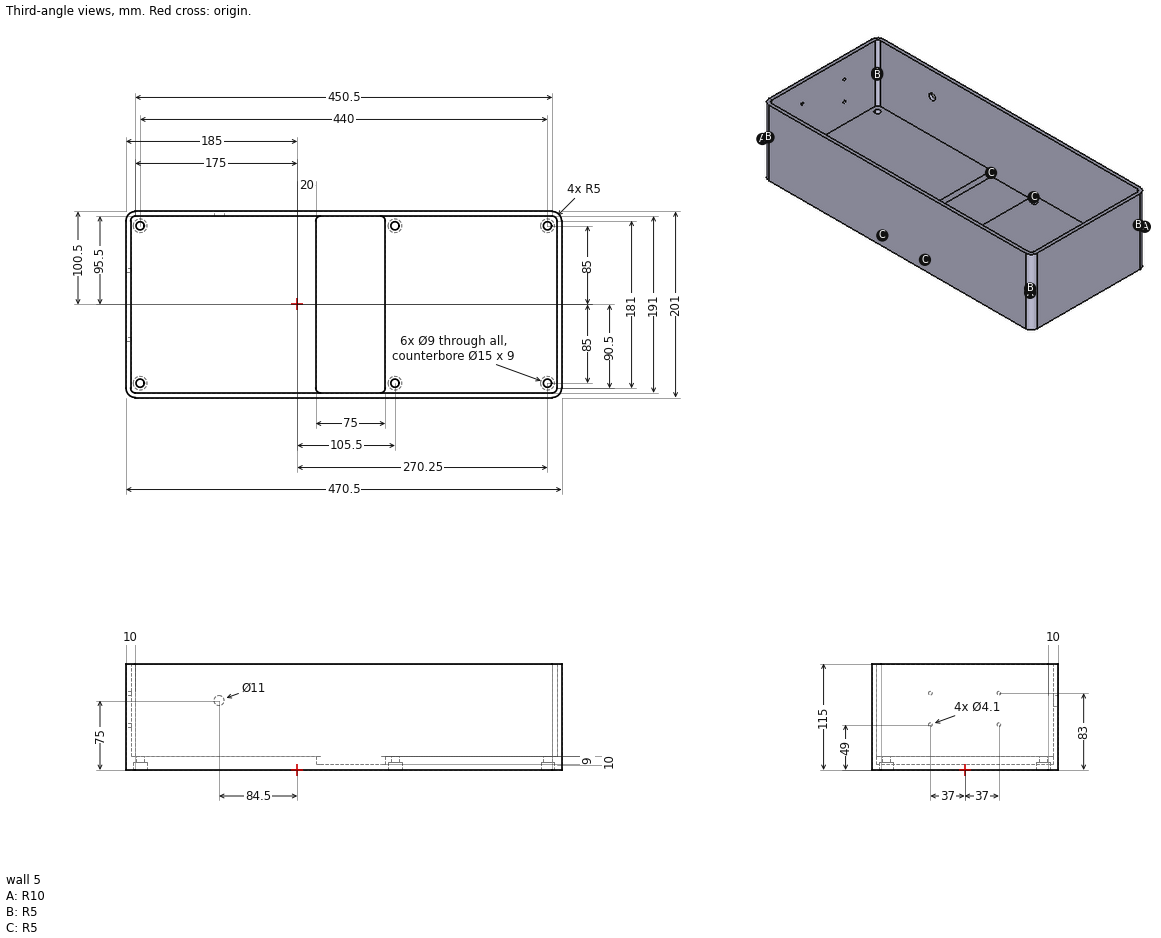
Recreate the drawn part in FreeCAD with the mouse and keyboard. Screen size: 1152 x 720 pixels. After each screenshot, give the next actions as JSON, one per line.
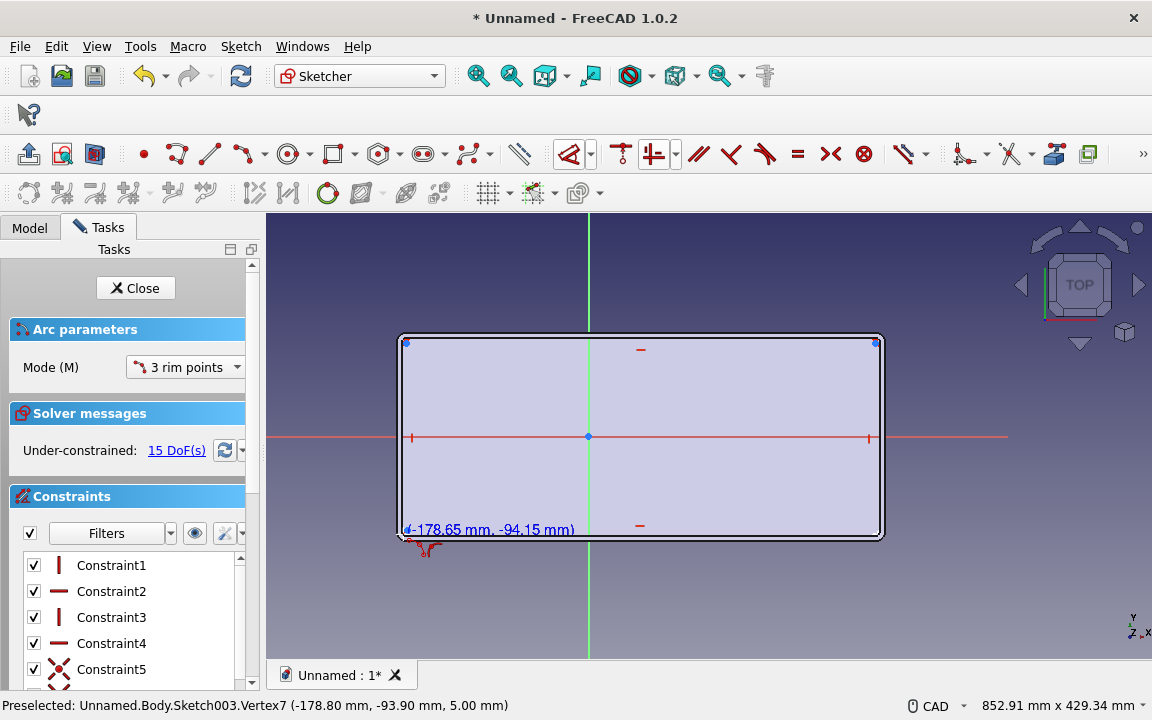
{"action": "scroll", "coordinate": [875, 536], "scroll_direction": "up", "scroll_amount": 4}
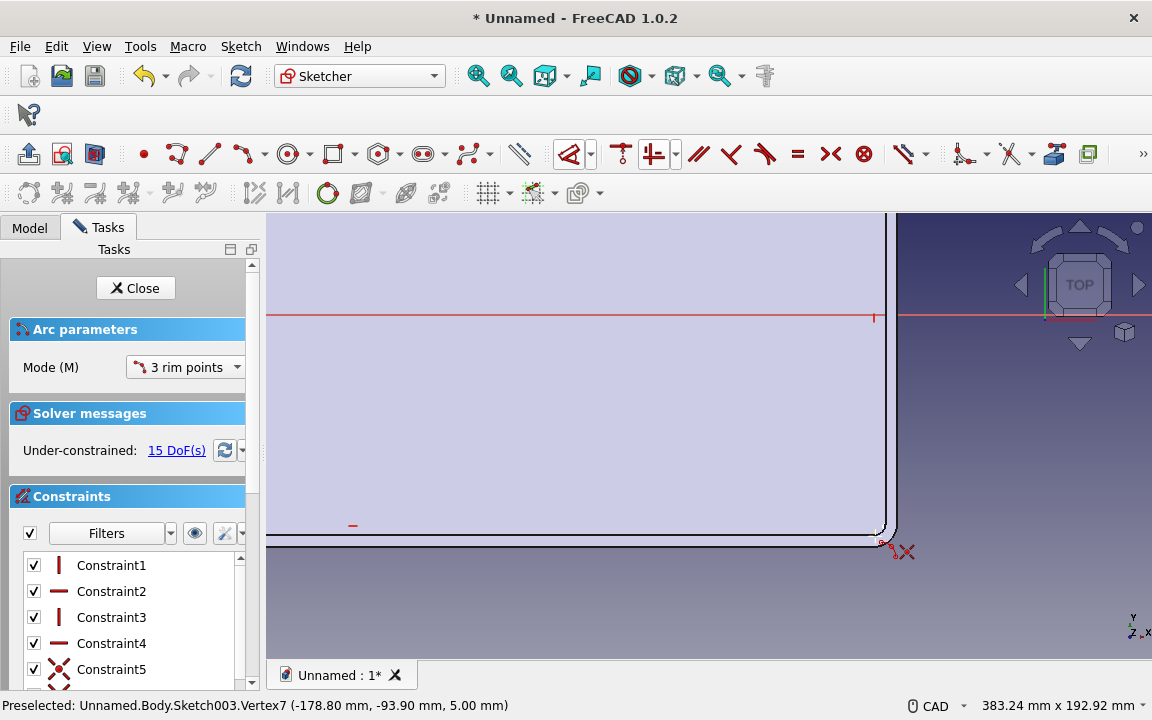
{"action": "left_click", "coordinate": [874, 536]}
{"action": "left_click", "coordinate": [886, 527]}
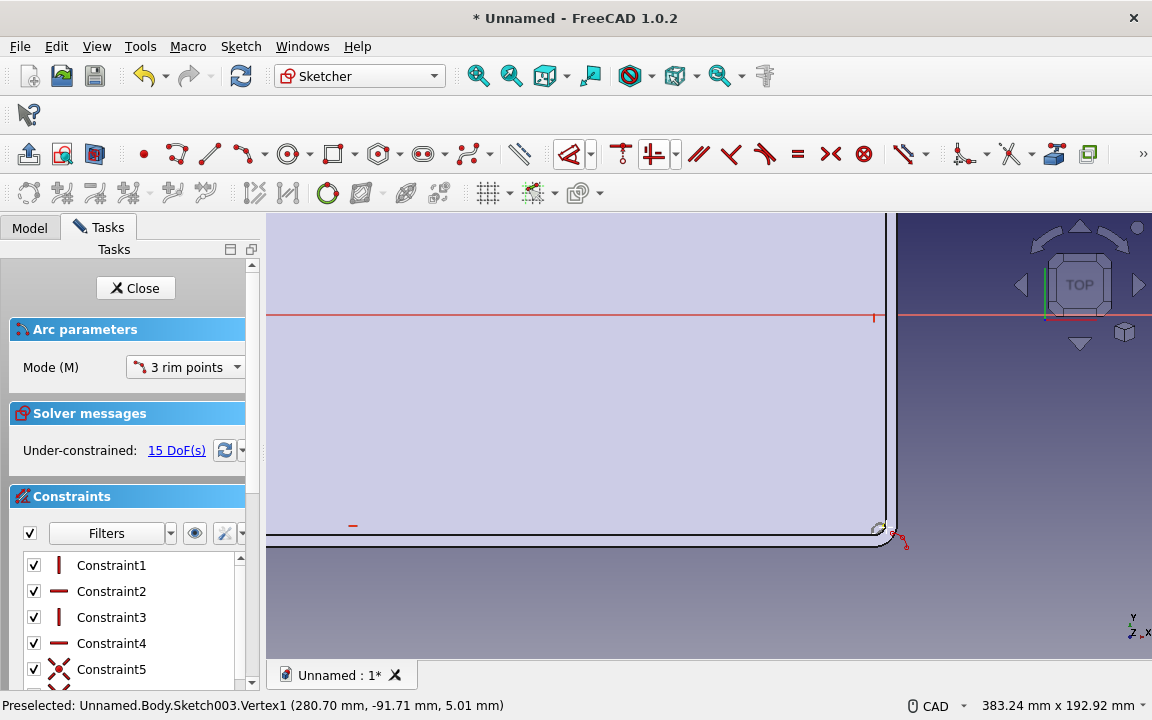
{"action": "scroll", "coordinate": [882, 532], "scroll_direction": "up", "scroll_amount": 8}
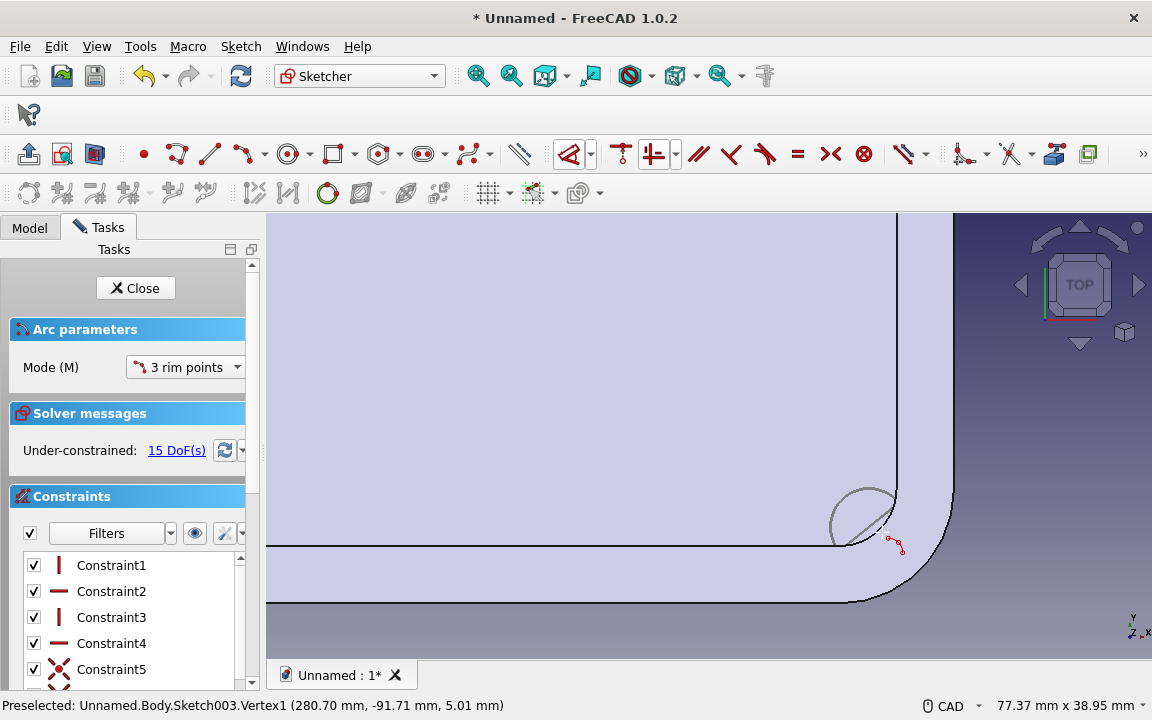
{"action": "left_click", "coordinate": [880, 529]}
{"action": "key", "text": "Escape"}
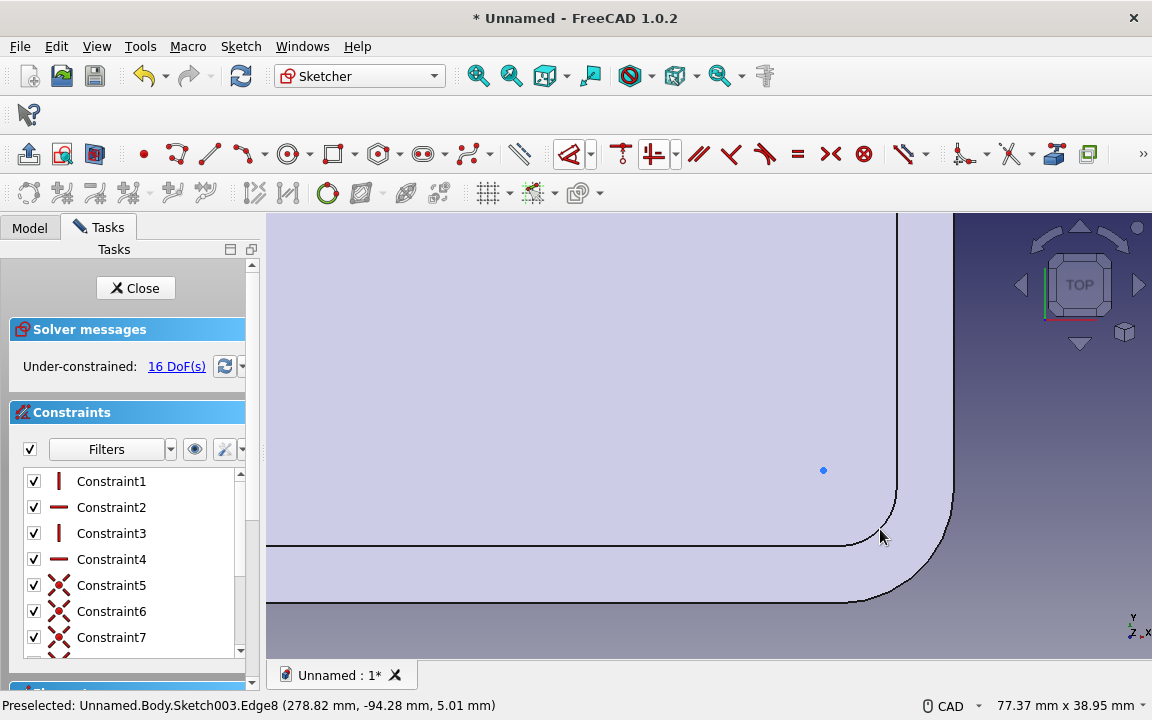
{"action": "scroll", "coordinate": [878, 534], "scroll_direction": "down", "scroll_amount": 12}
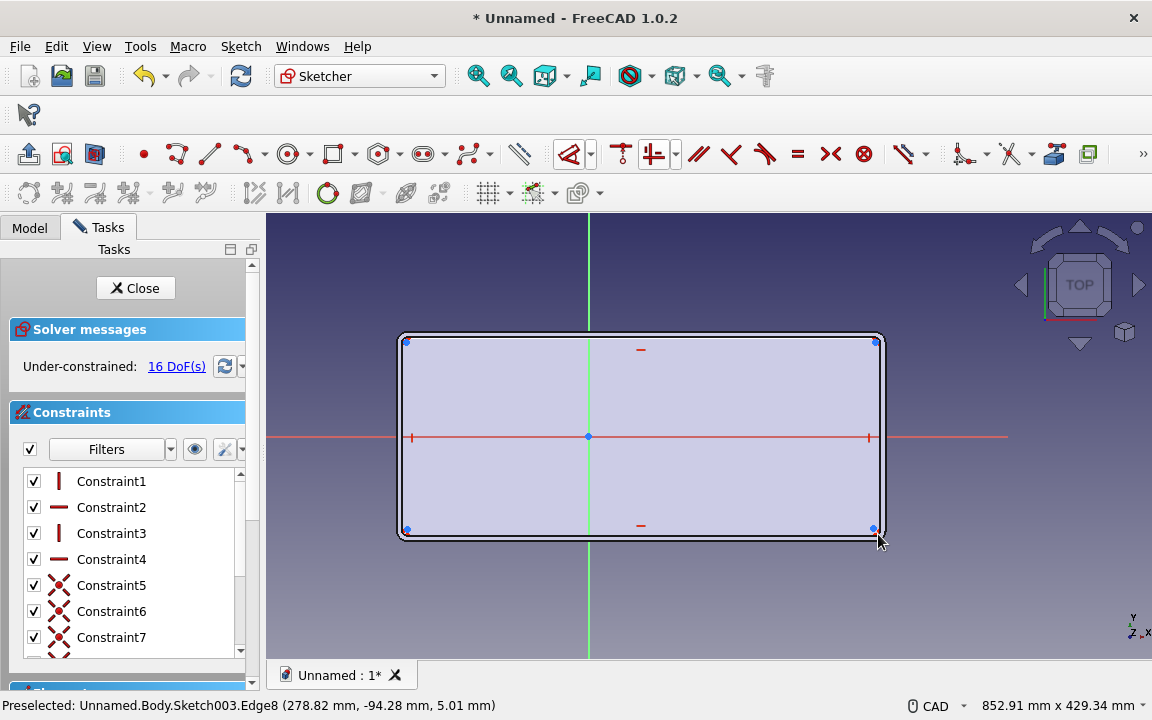
{"action": "left_click", "coordinate": [881, 475]}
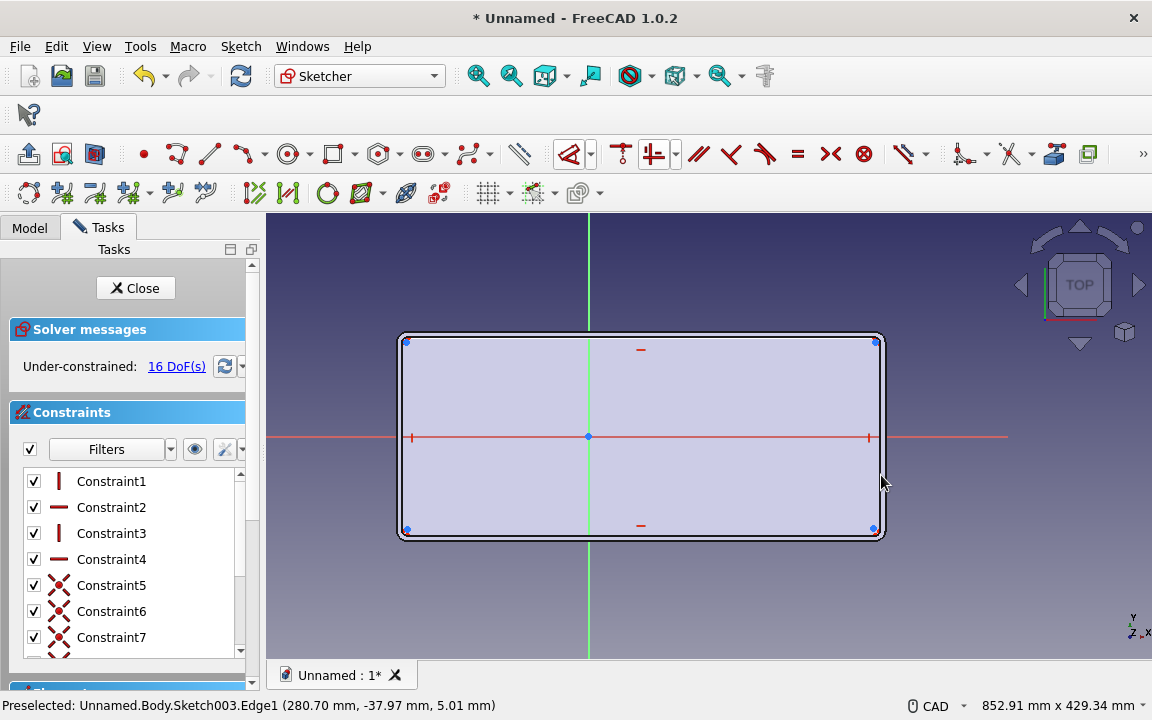
{"action": "scroll", "coordinate": [879, 339], "scroll_direction": "up", "scroll_amount": 6}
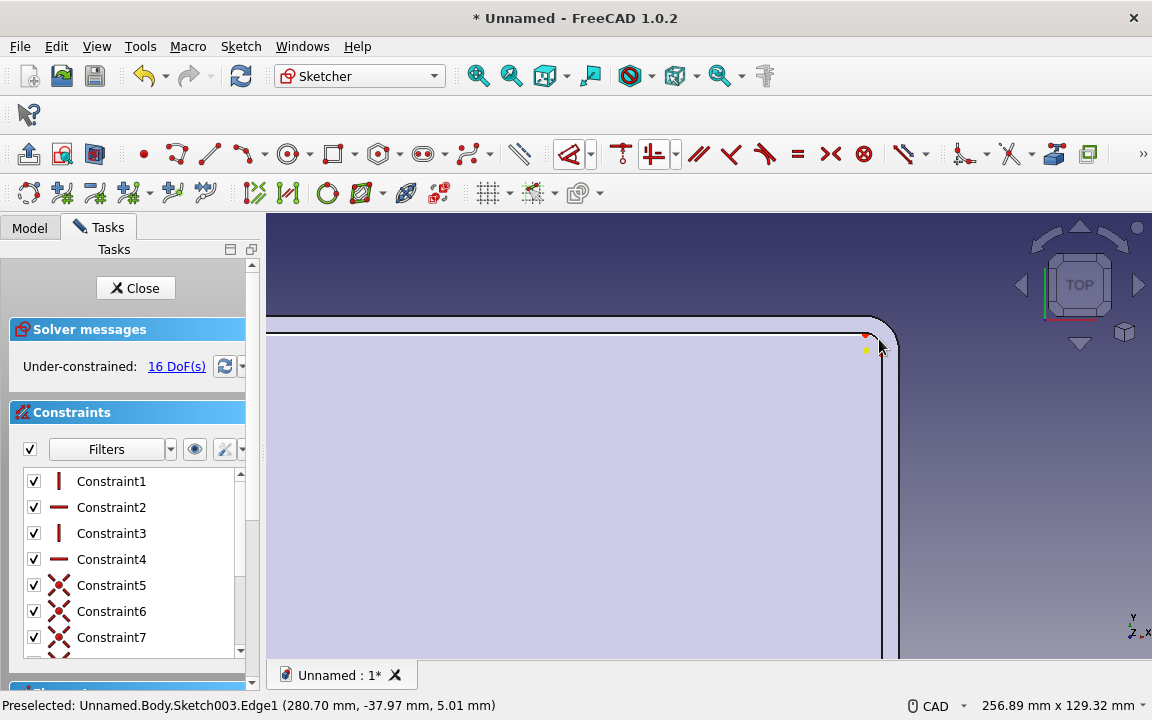
{"action": "left_click", "coordinate": [879, 340]}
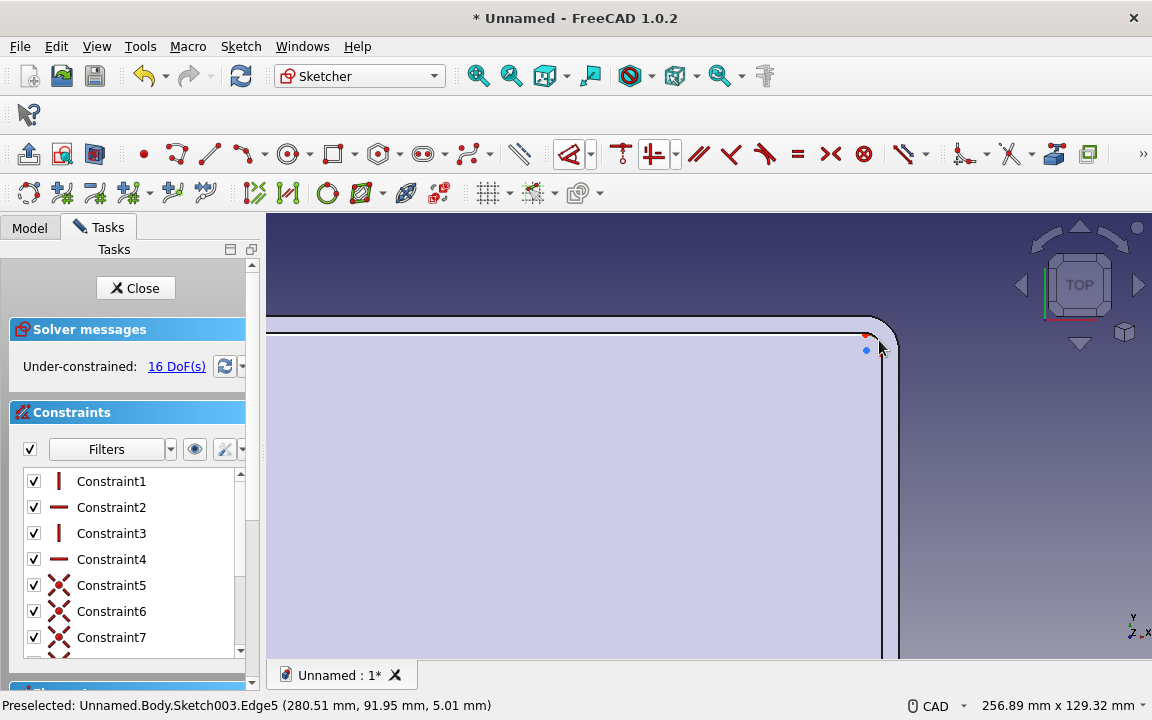
{"action": "key", "text": "t"}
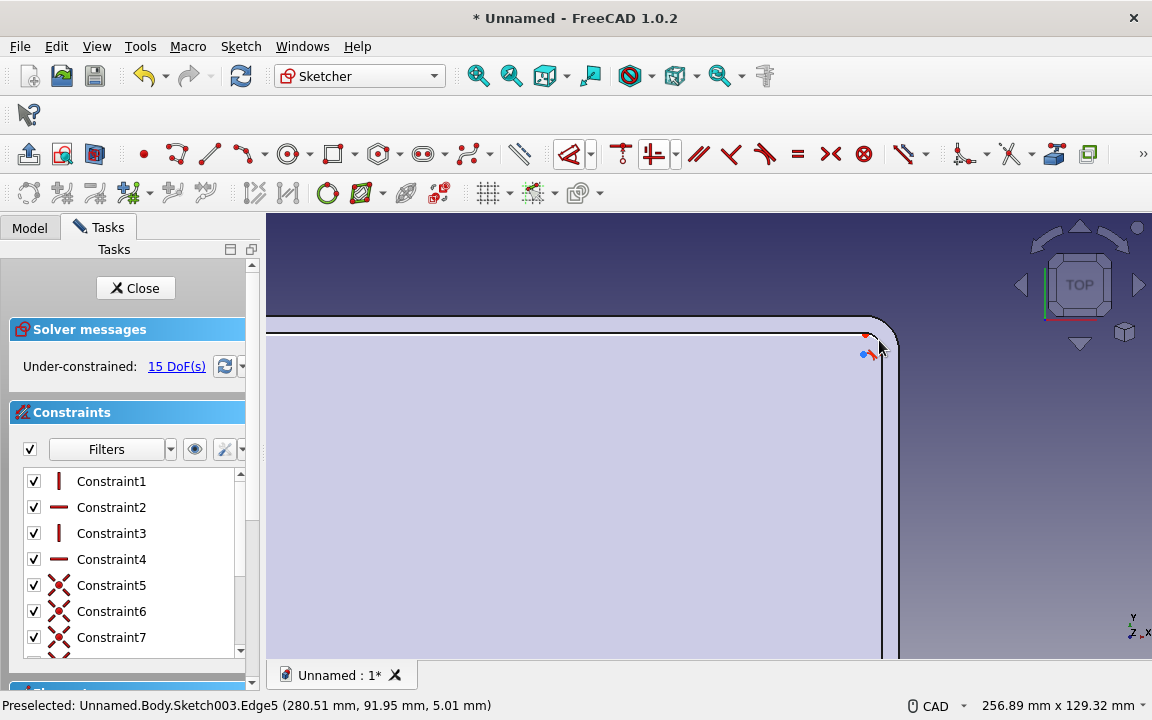
{"action": "scroll", "coordinate": [879, 338], "scroll_direction": "down", "scroll_amount": 6}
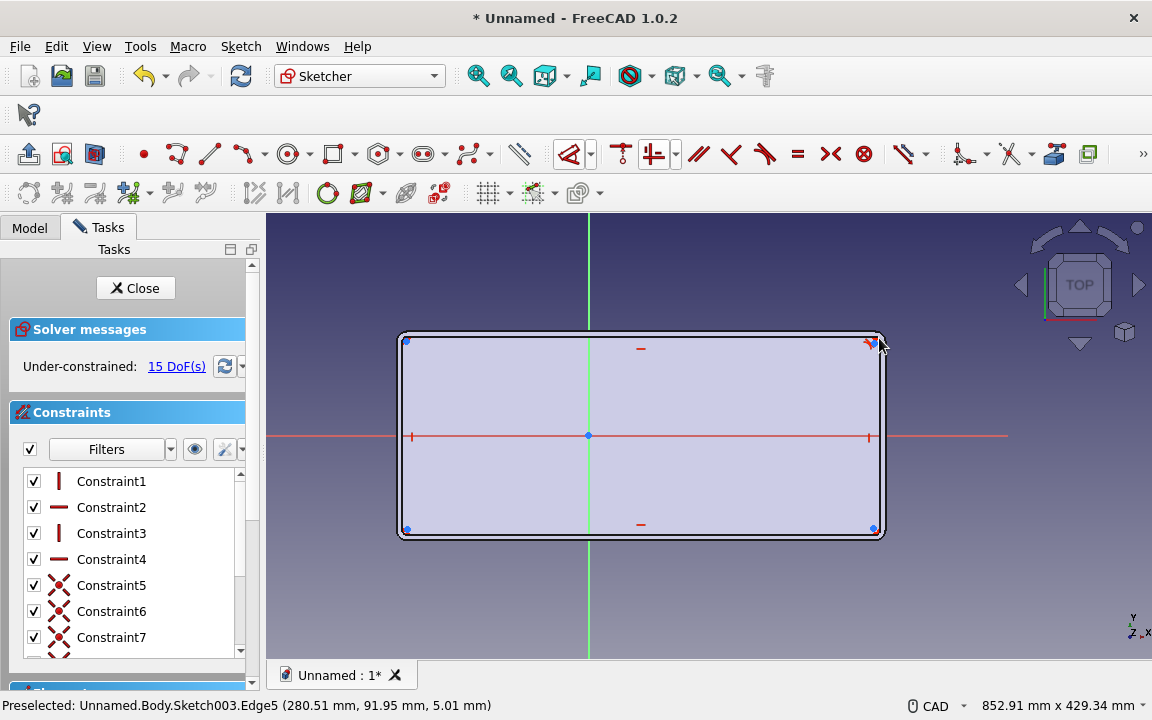
{"action": "left_click", "coordinate": [881, 399]}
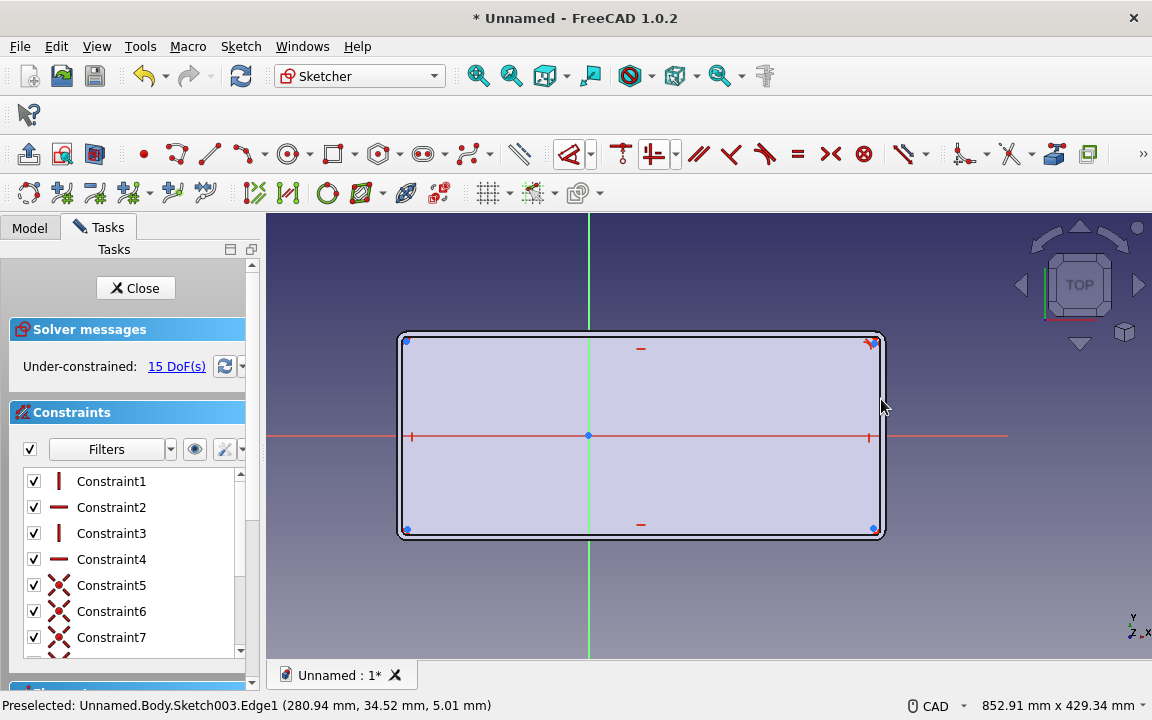
{"action": "scroll", "coordinate": [879, 534], "scroll_direction": "up", "scroll_amount": 7}